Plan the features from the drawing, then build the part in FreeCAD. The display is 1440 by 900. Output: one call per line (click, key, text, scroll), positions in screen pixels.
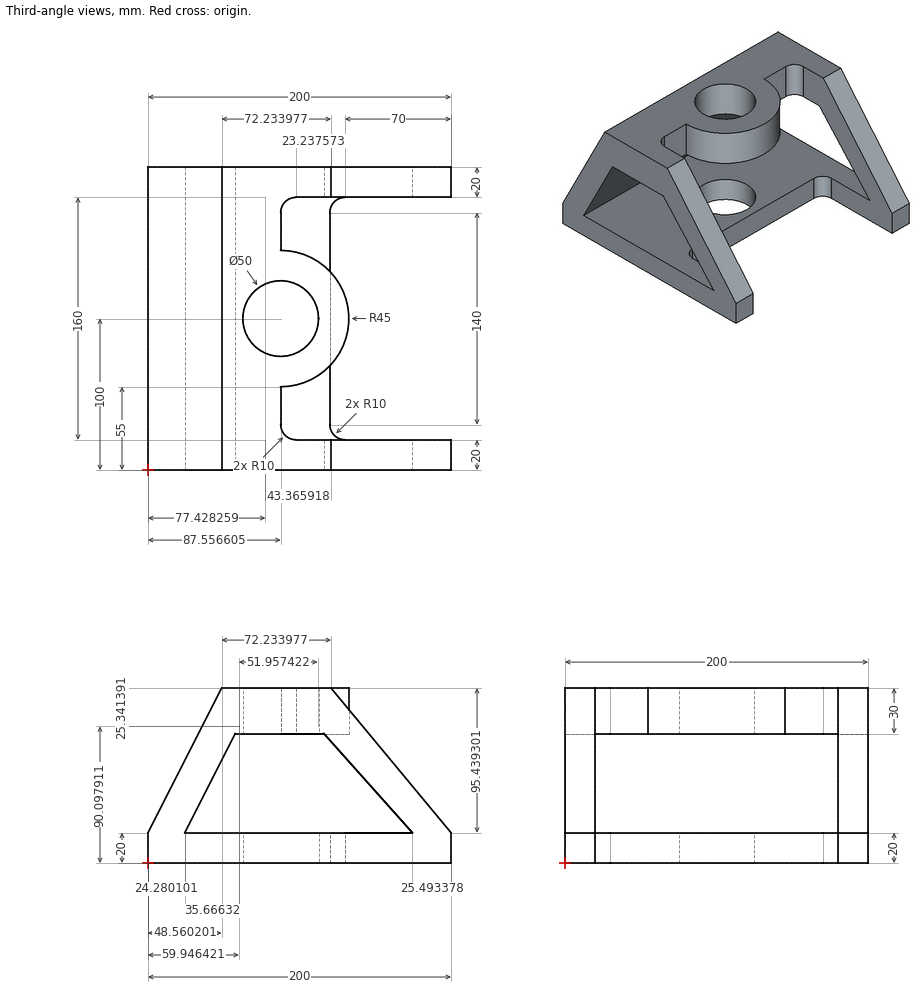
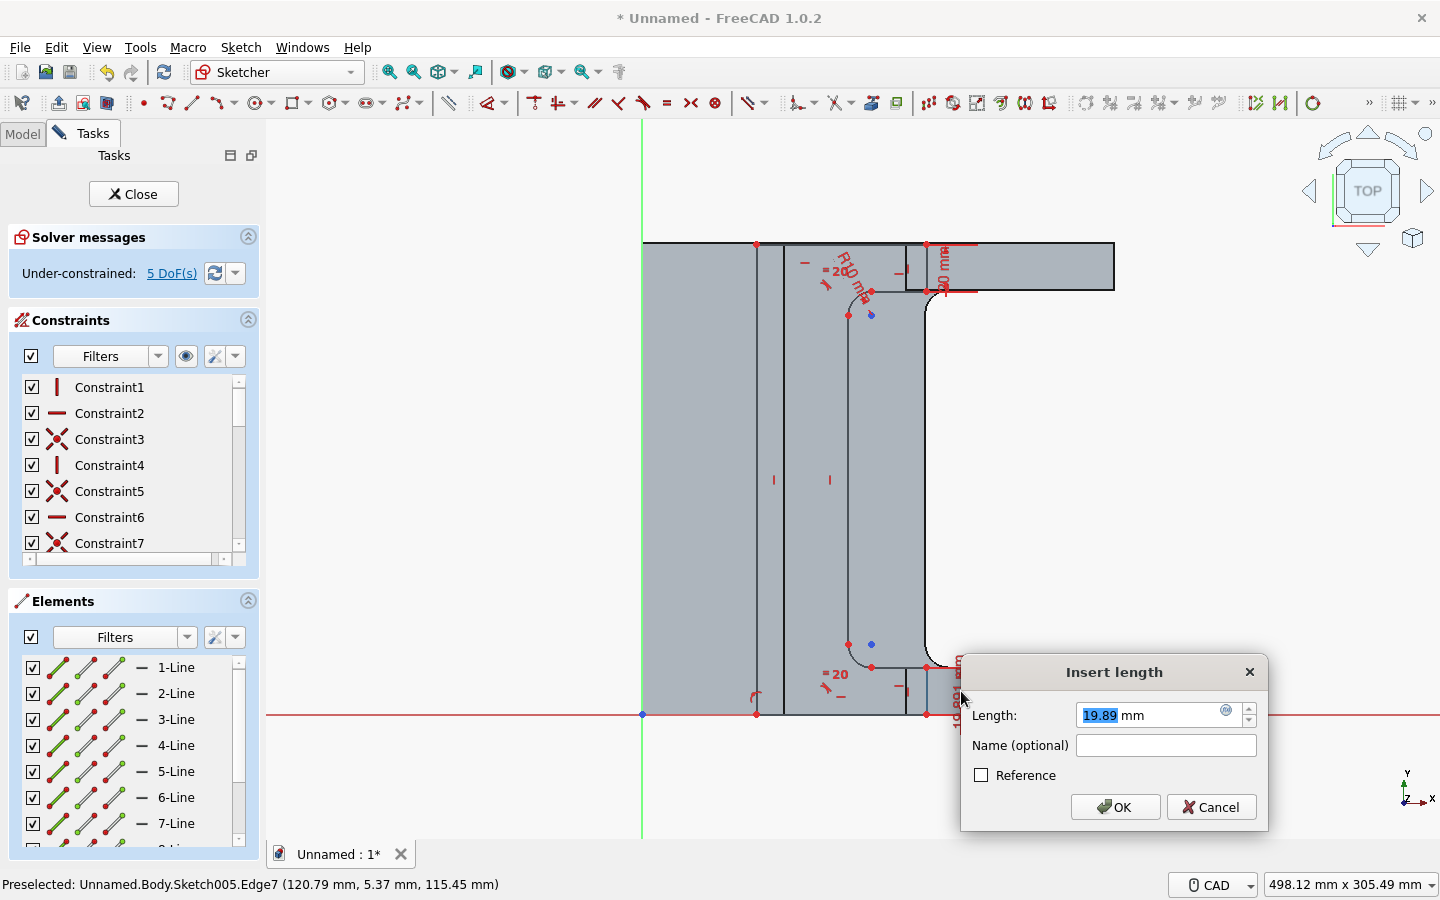
text(20)
key(Return)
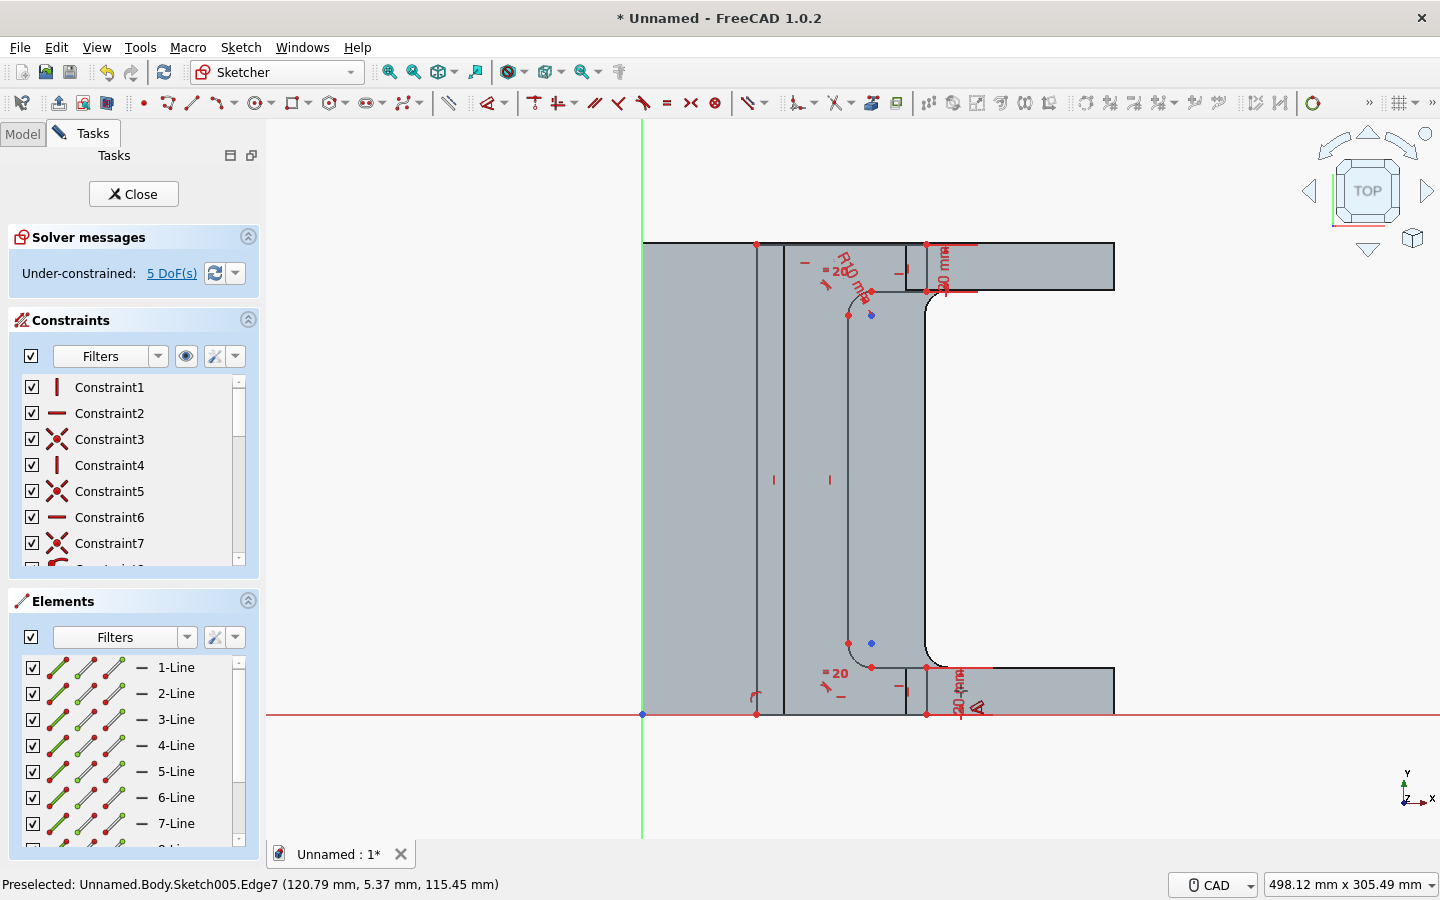
click(848, 545)
click(882, 480)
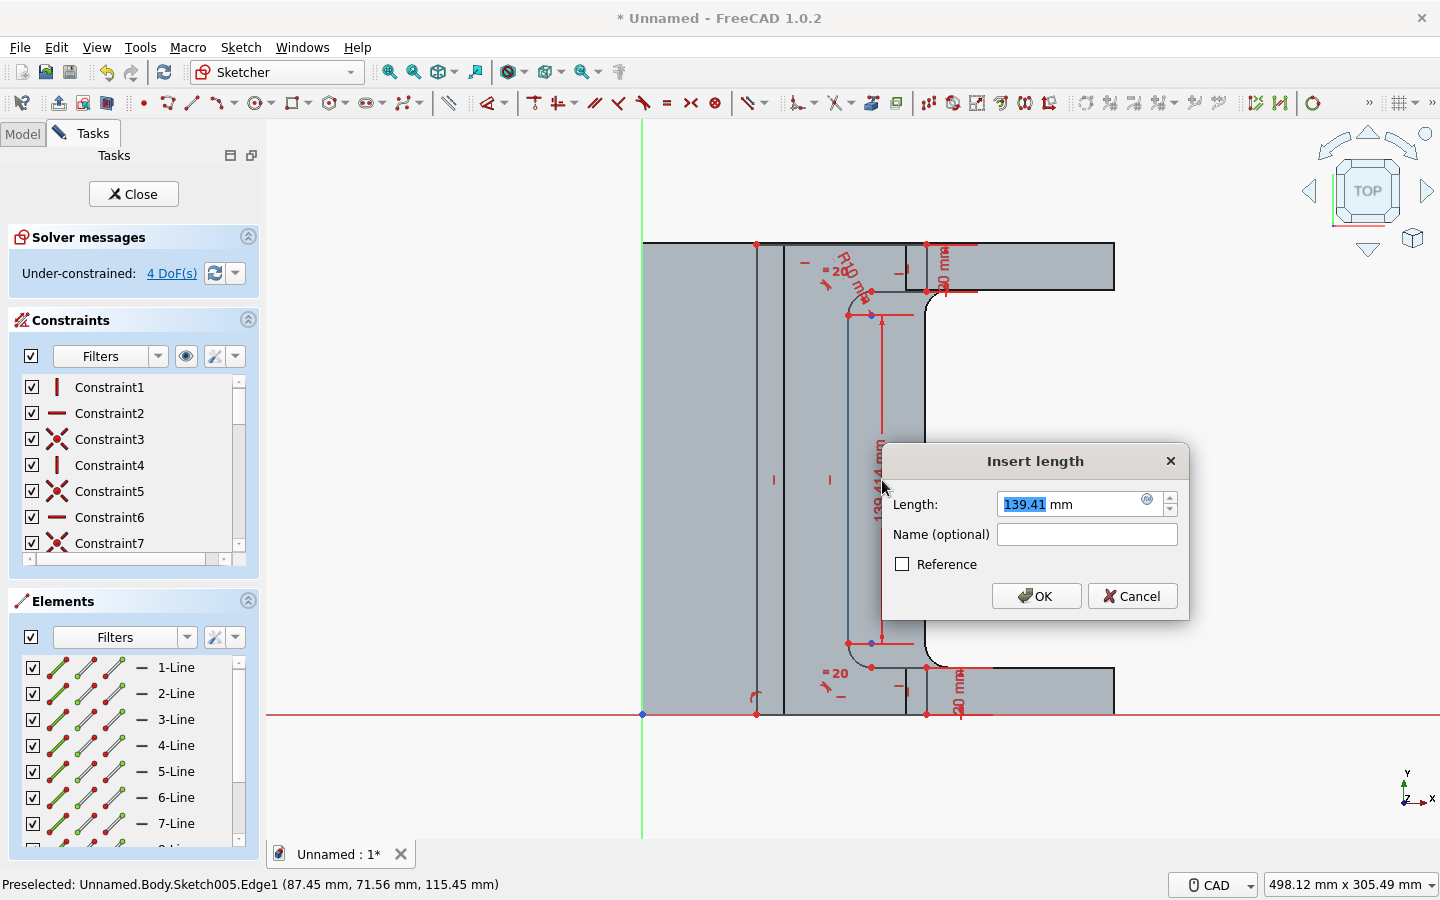
text(140)
key(Return)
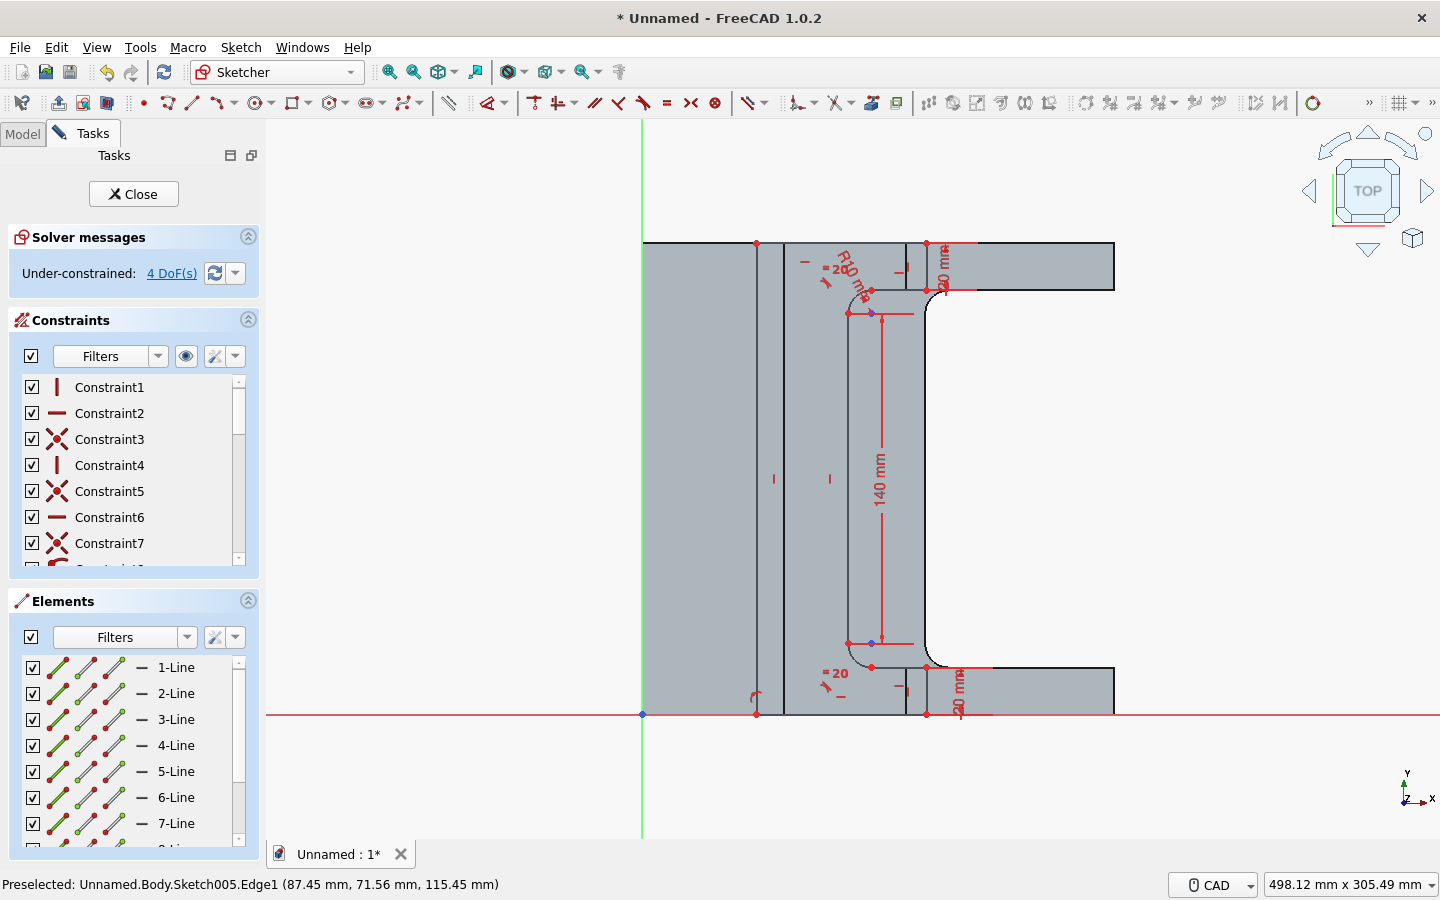
click(888, 290)
click(899, 324)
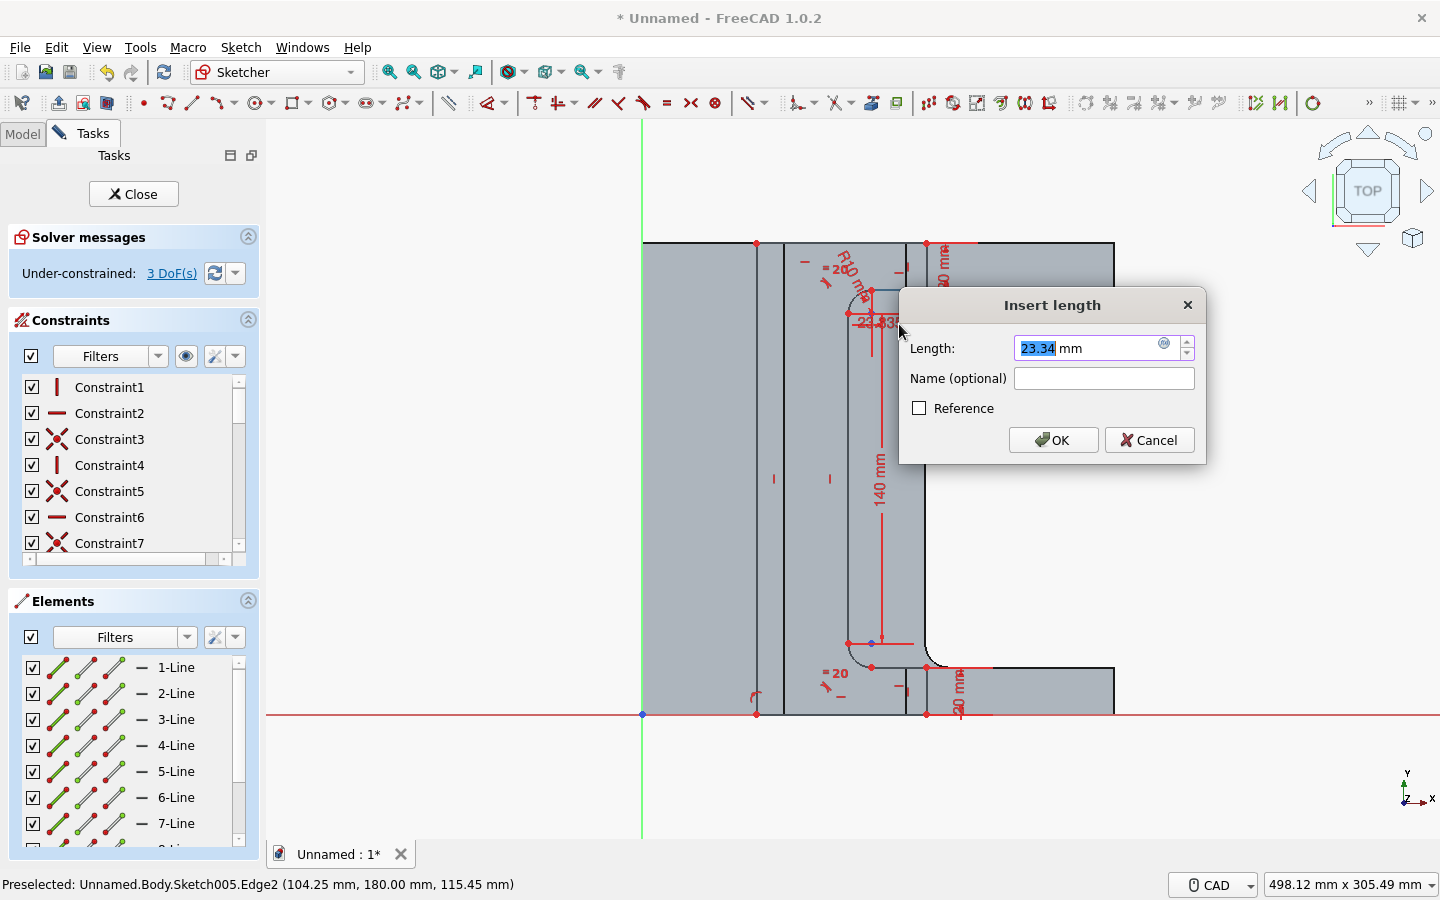
text(23.237573)
key(Return)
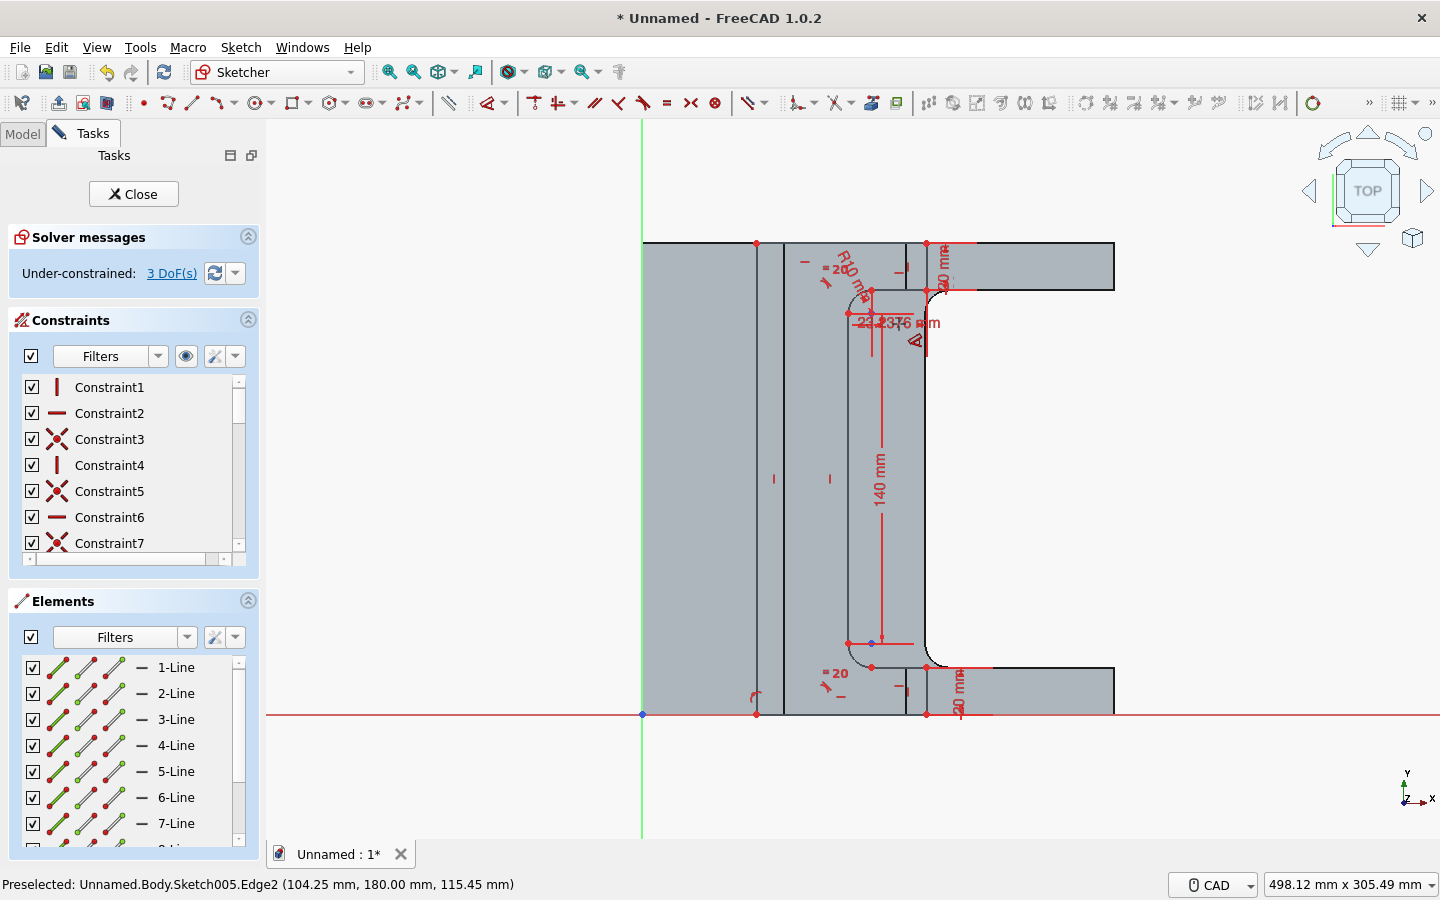
click(876, 243)
click(842, 209)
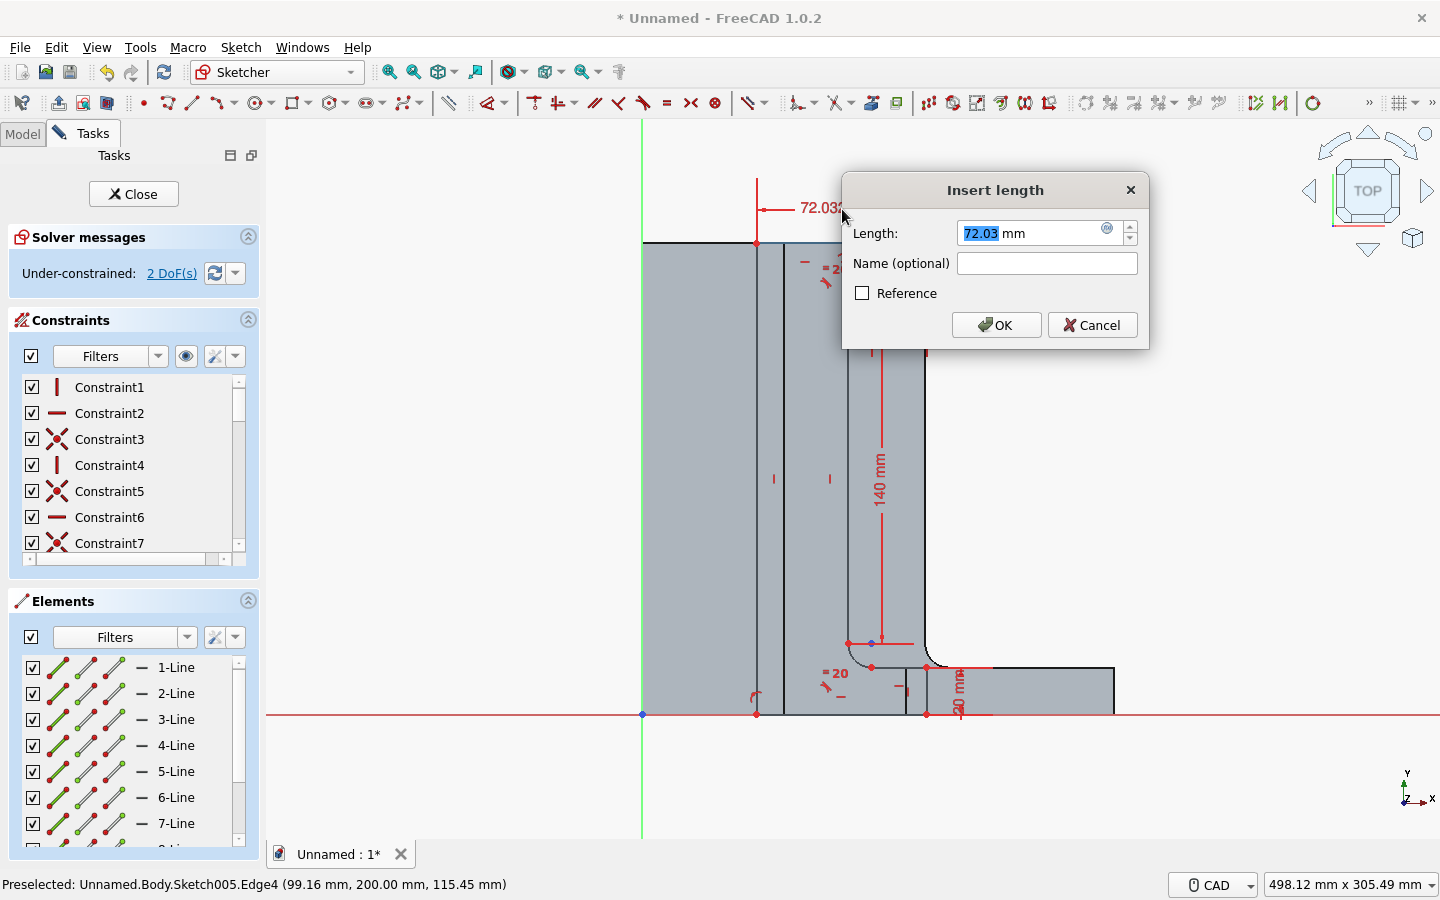
text(72.233977)
key(Return)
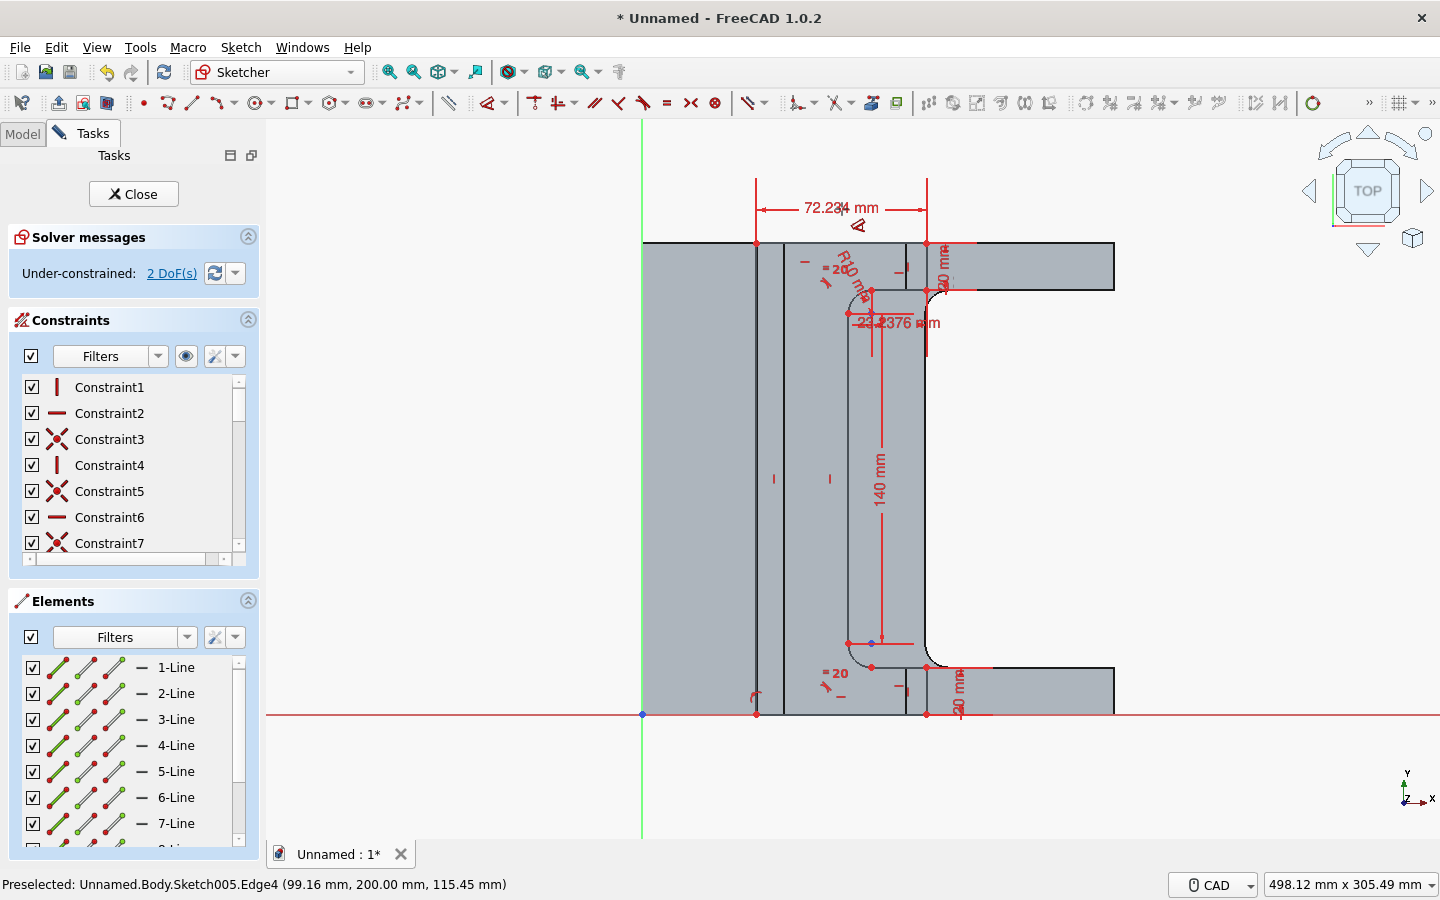
click(808, 715)
click(842, 749)